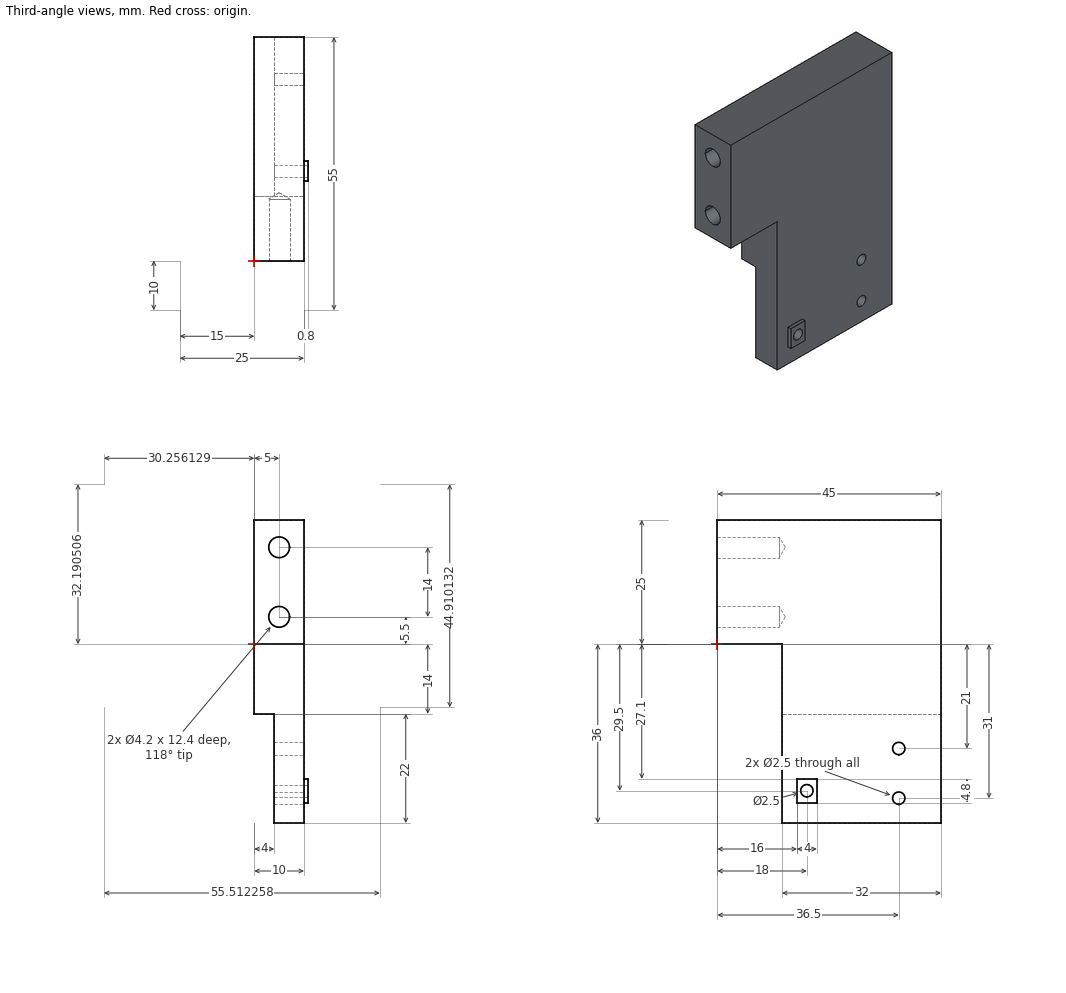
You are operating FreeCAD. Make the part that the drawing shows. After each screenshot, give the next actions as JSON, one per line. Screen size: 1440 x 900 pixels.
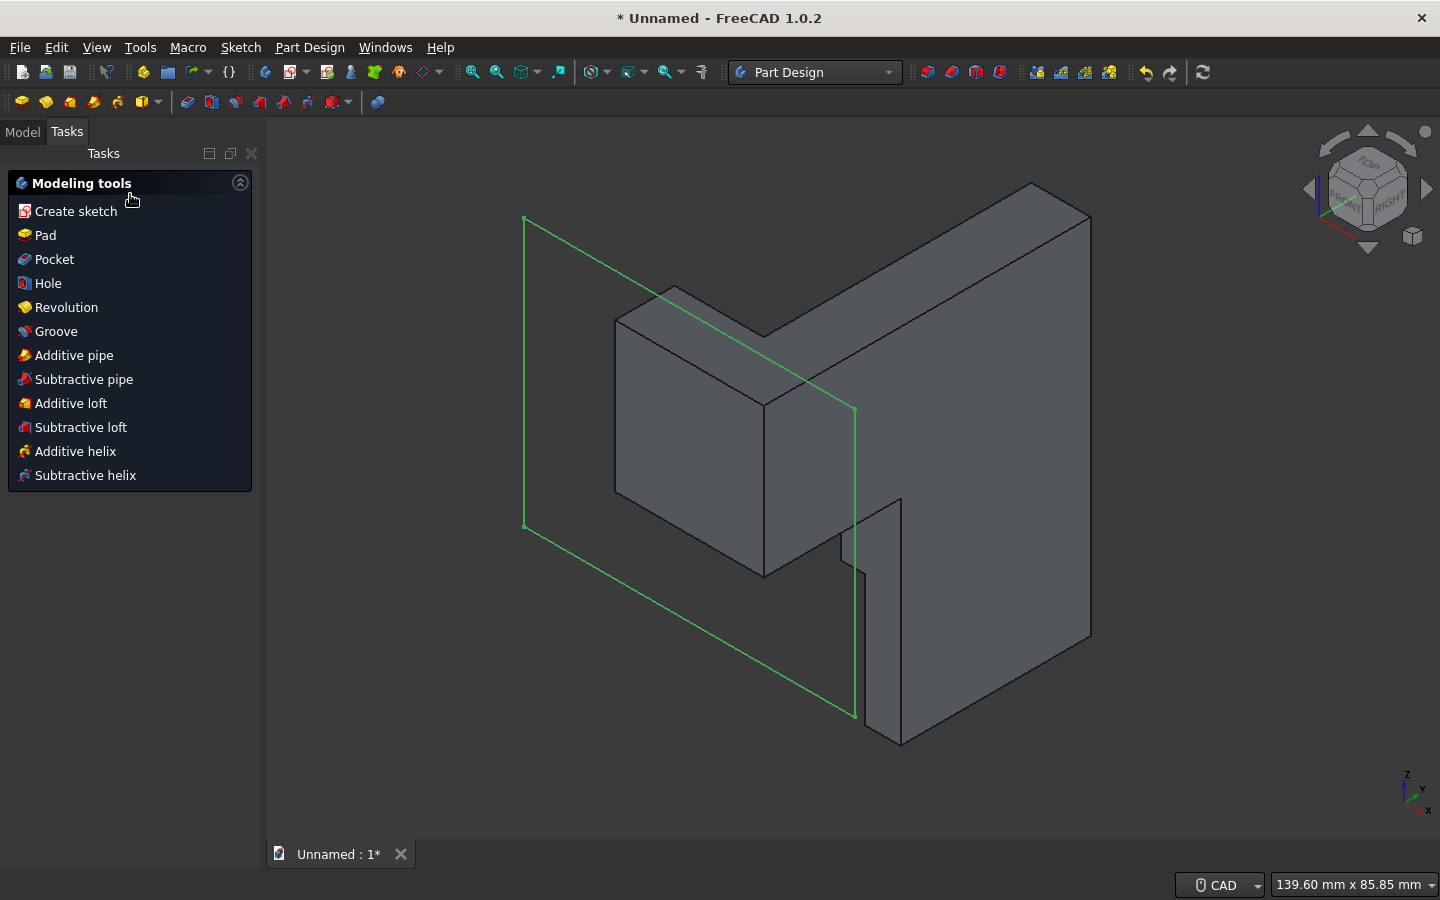
{"action": "left_click", "coordinate": [188, 102]}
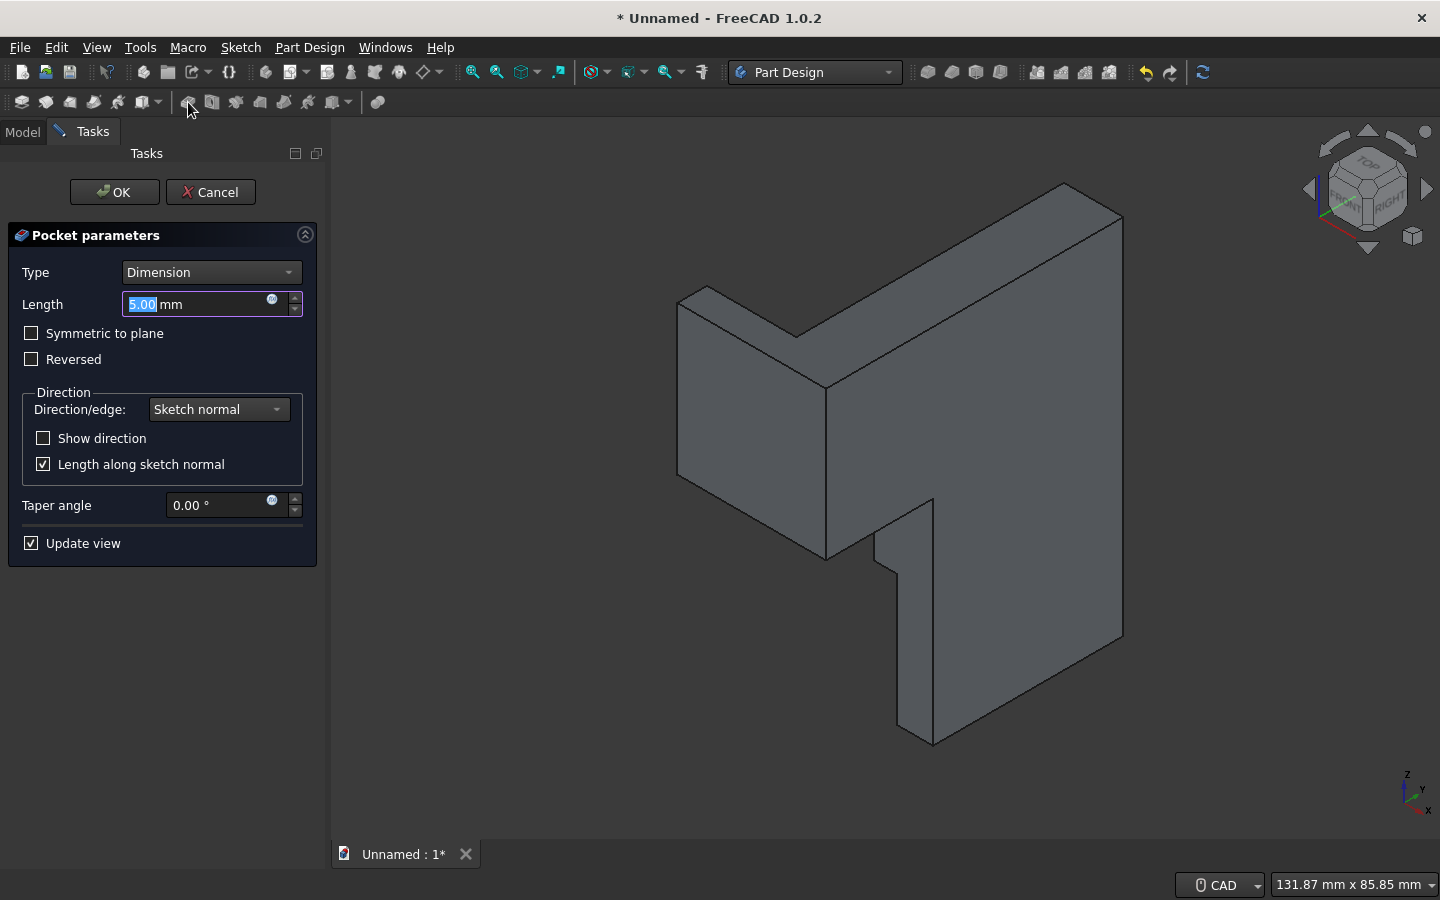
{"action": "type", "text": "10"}
{"action": "key", "text": "Tab"}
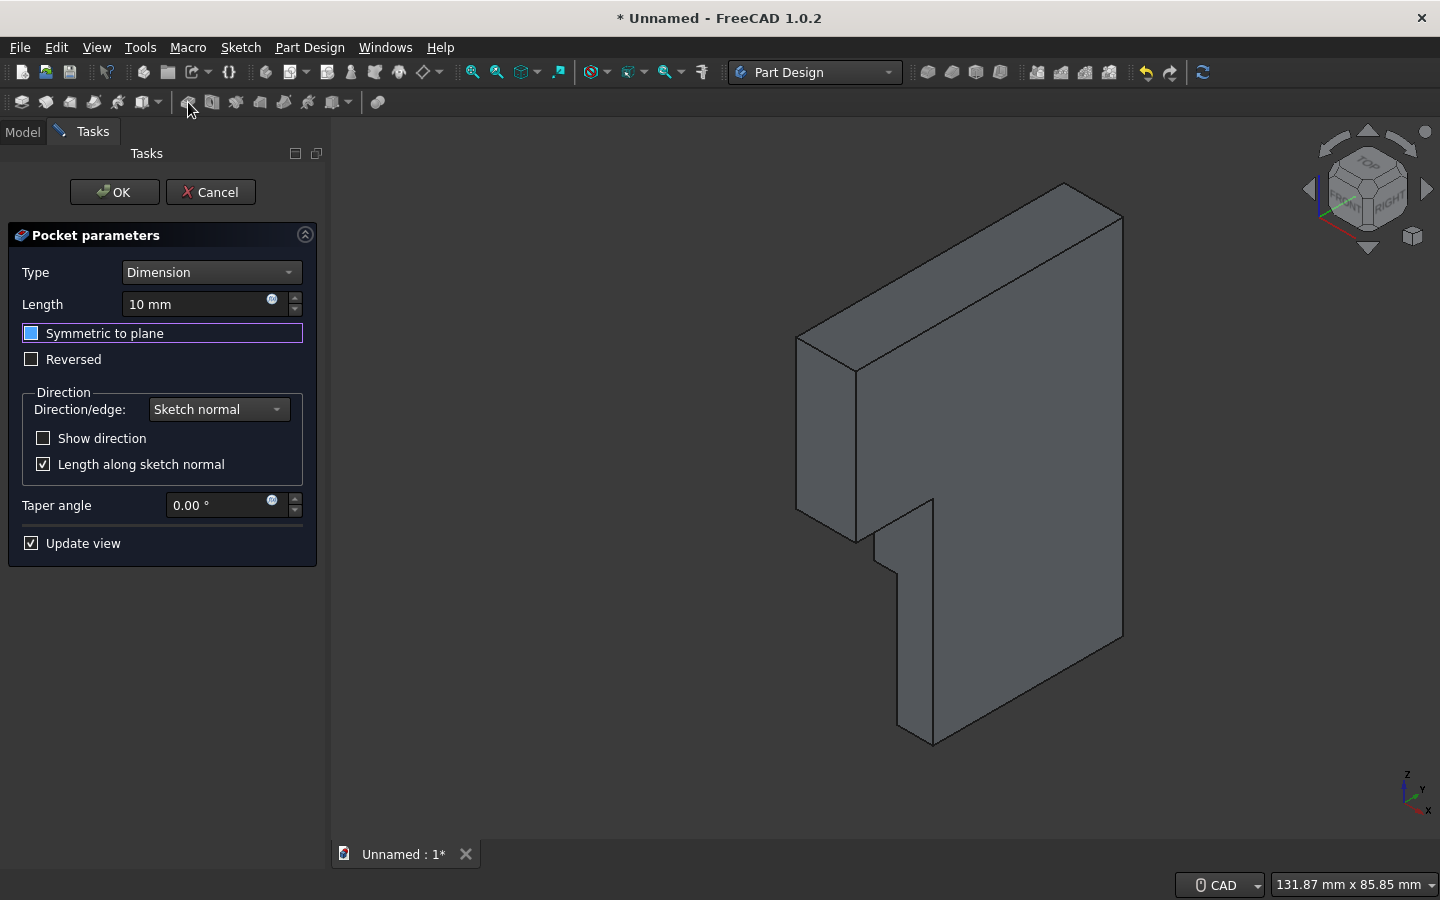
{"action": "left_click", "coordinate": [115, 192]}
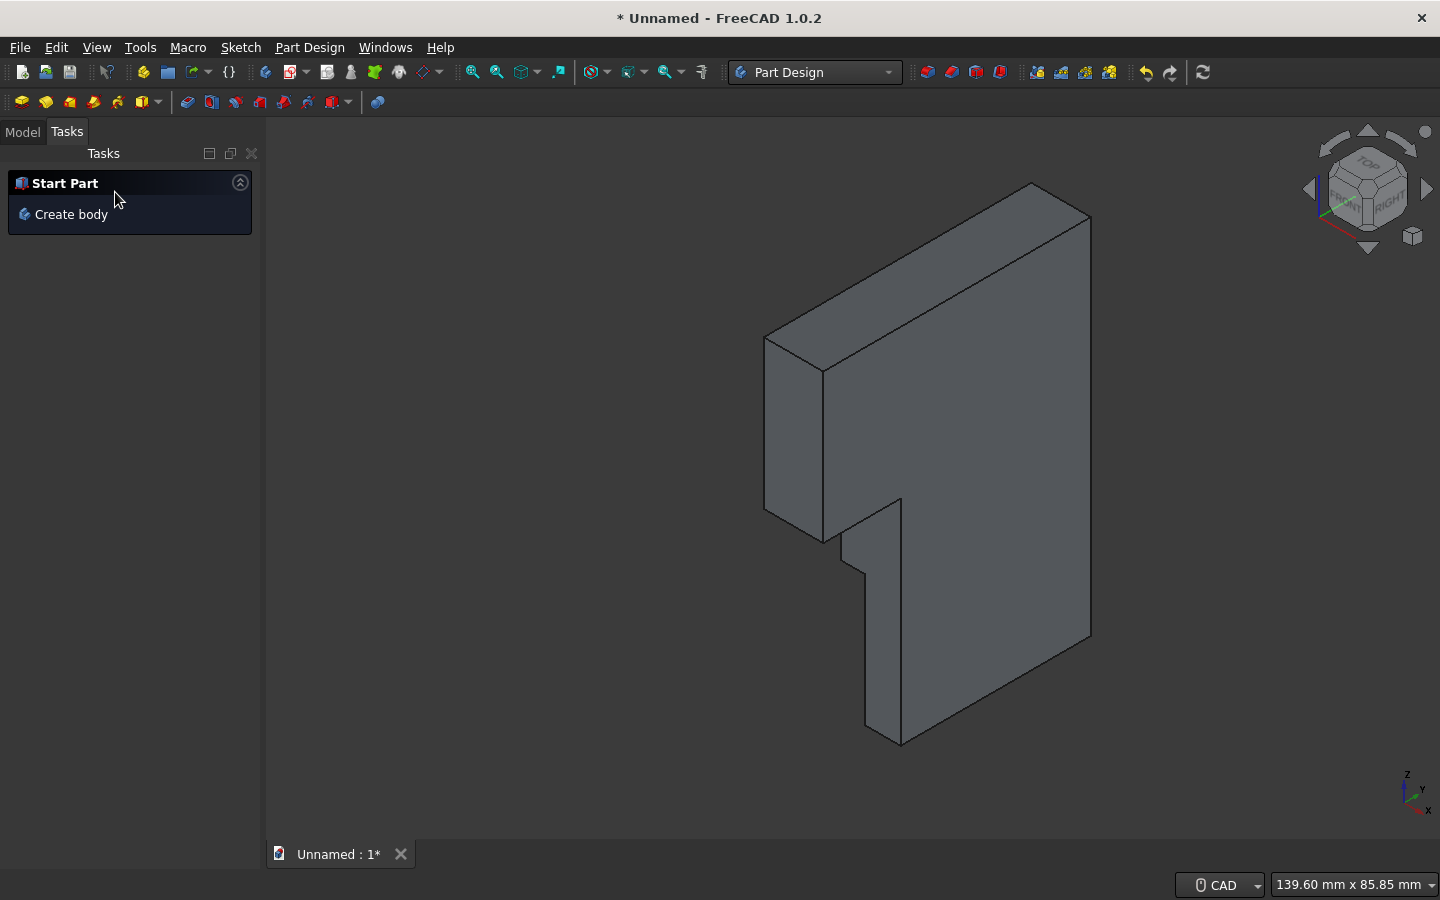
{"action": "left_click", "coordinate": [290, 72]}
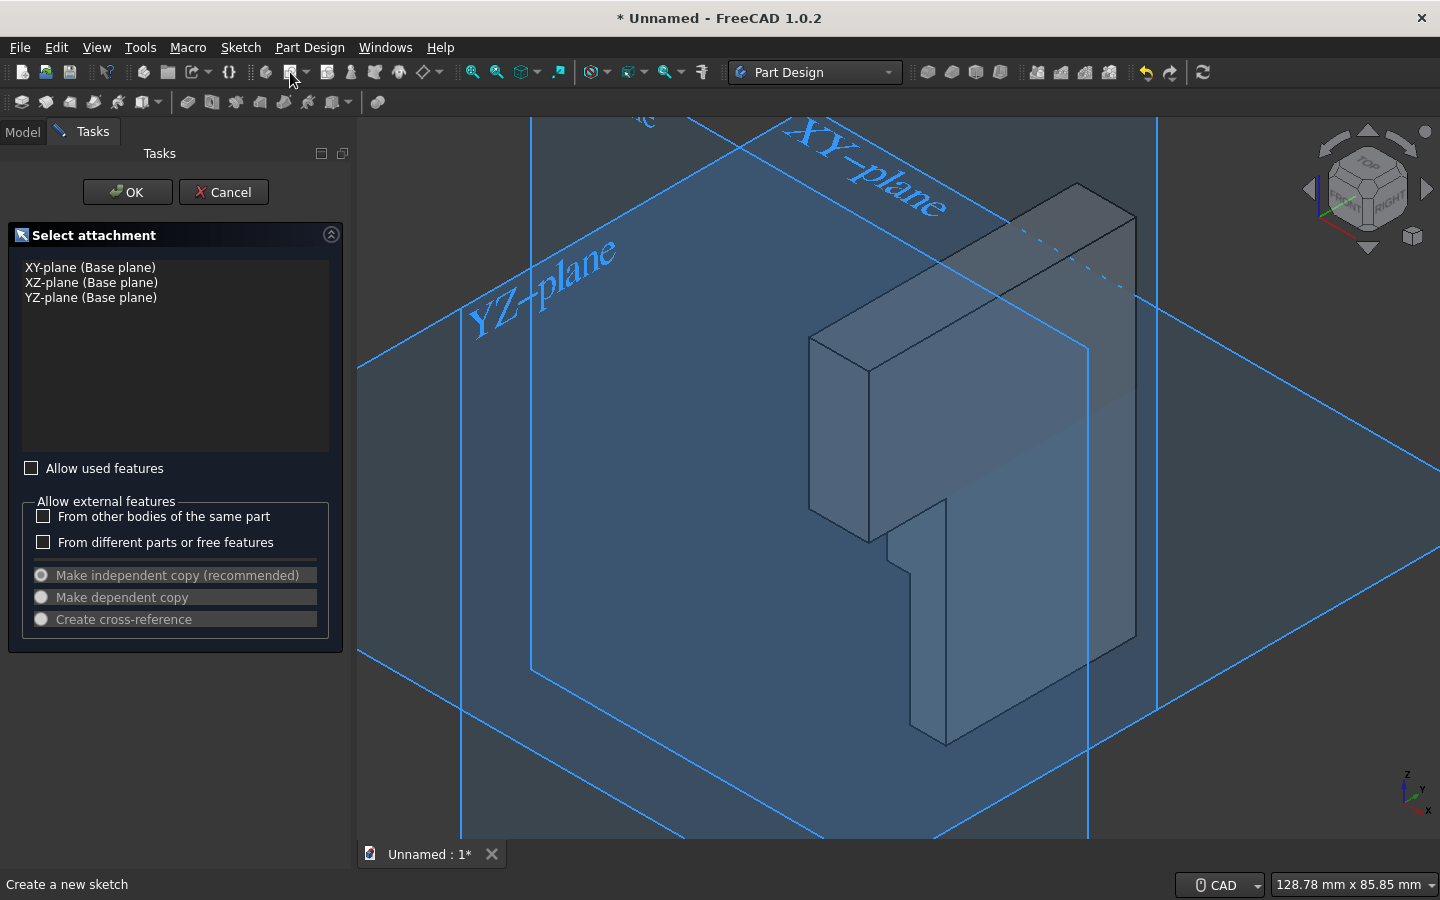
{"action": "left_click", "coordinate": [82, 282]}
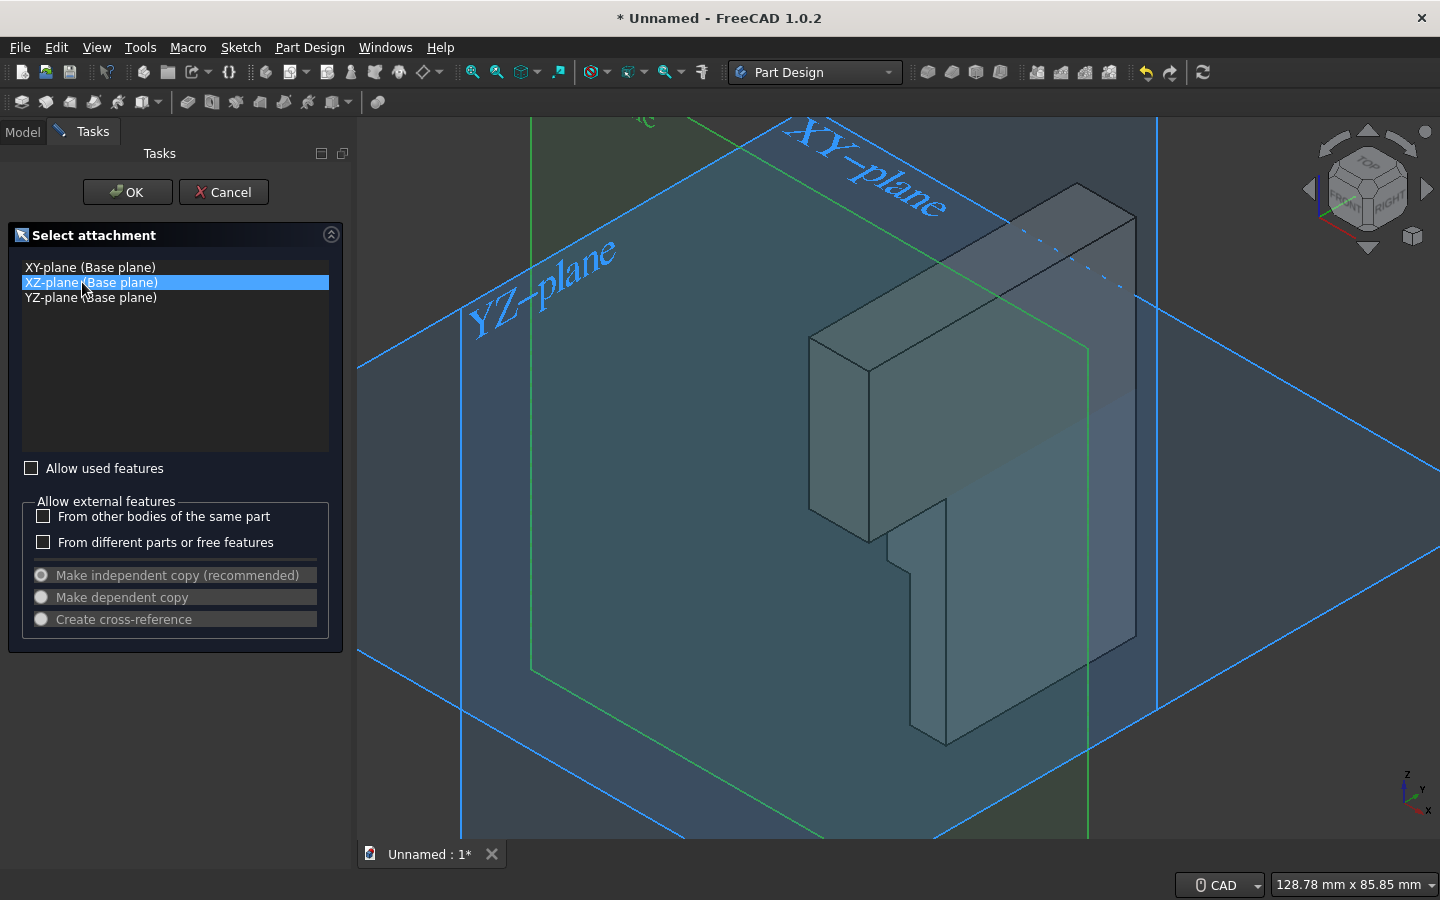
{"action": "left_click", "coordinate": [128, 192]}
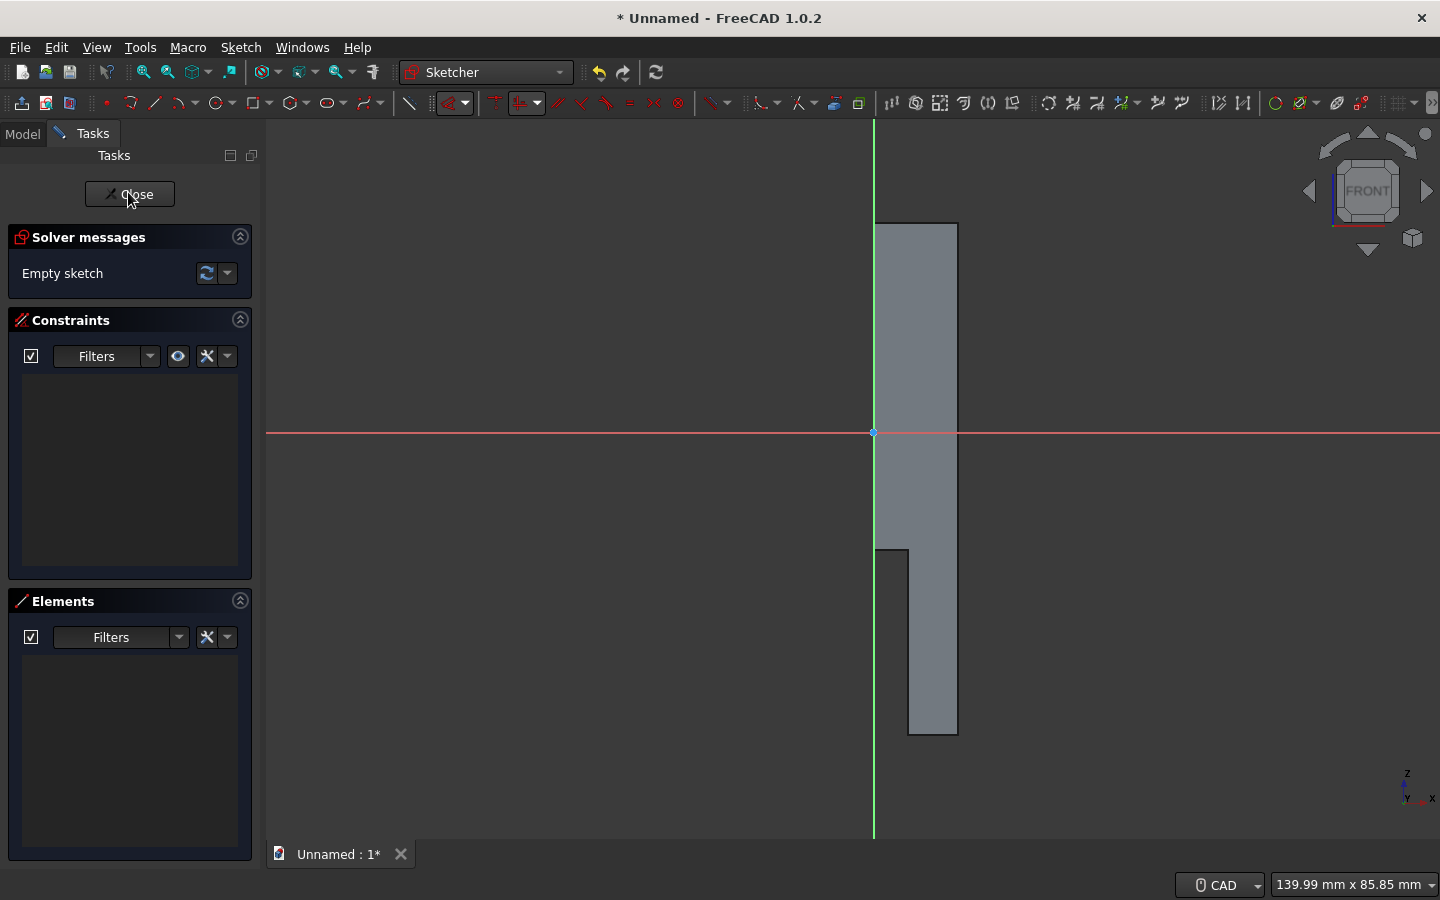
{"action": "scroll", "coordinate": [973, 263], "scroll_direction": "up", "scroll_amount": 5}